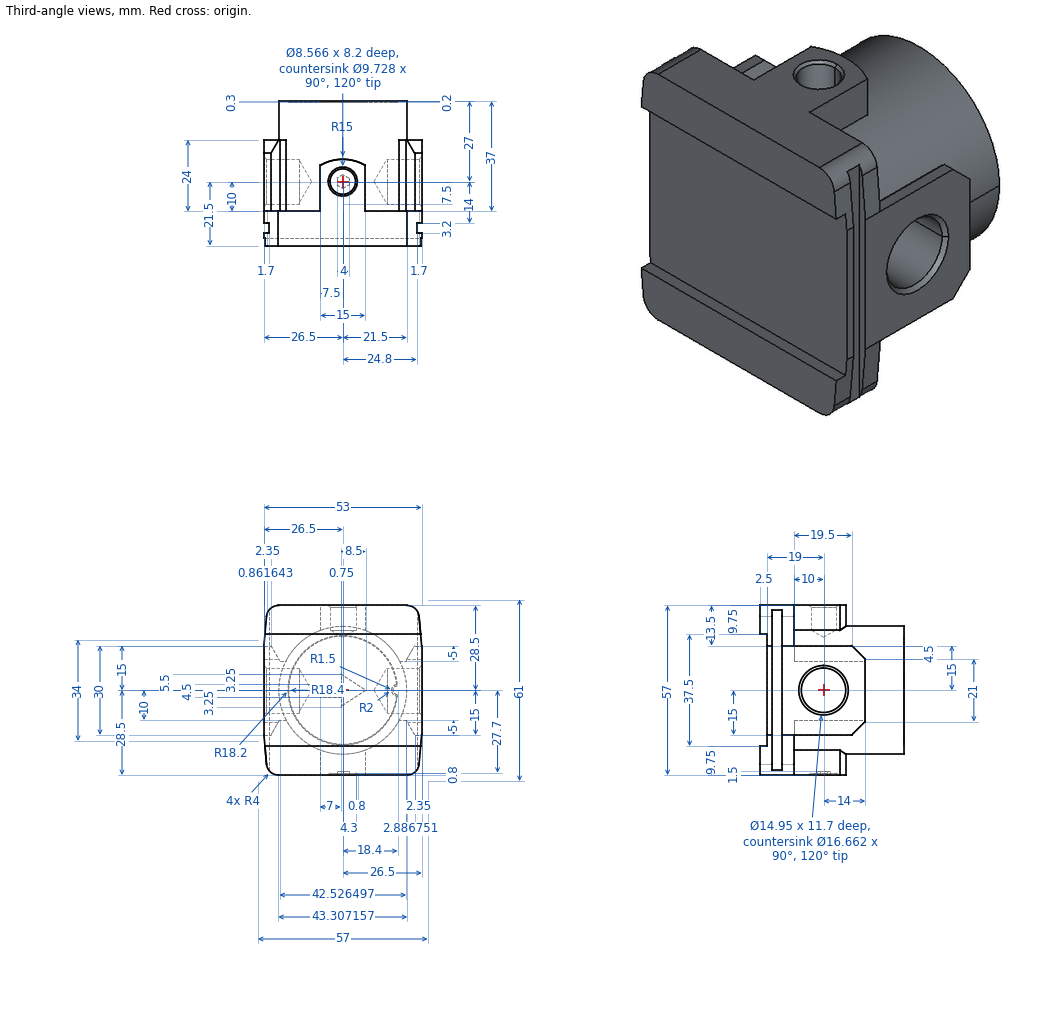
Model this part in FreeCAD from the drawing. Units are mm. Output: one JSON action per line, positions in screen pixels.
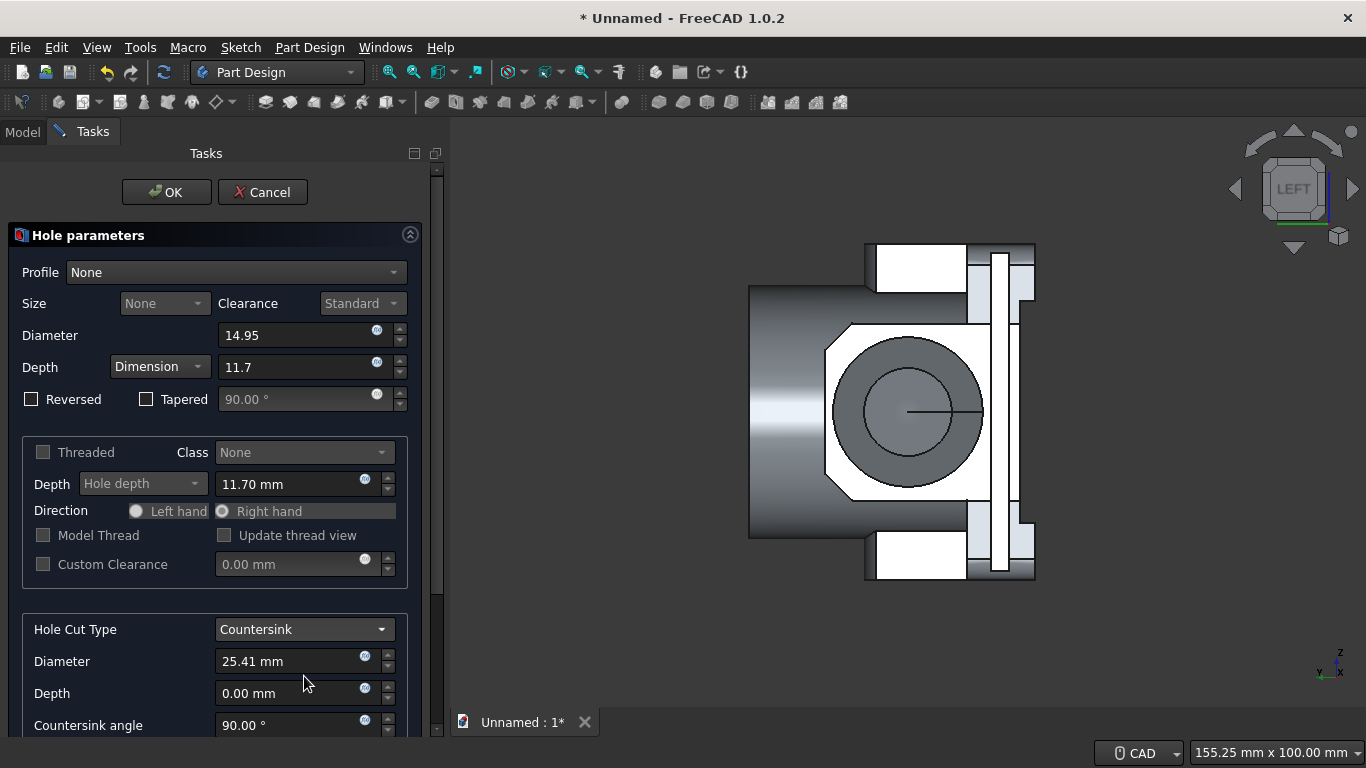
{"action": "triple_click", "coordinate": [298, 661]}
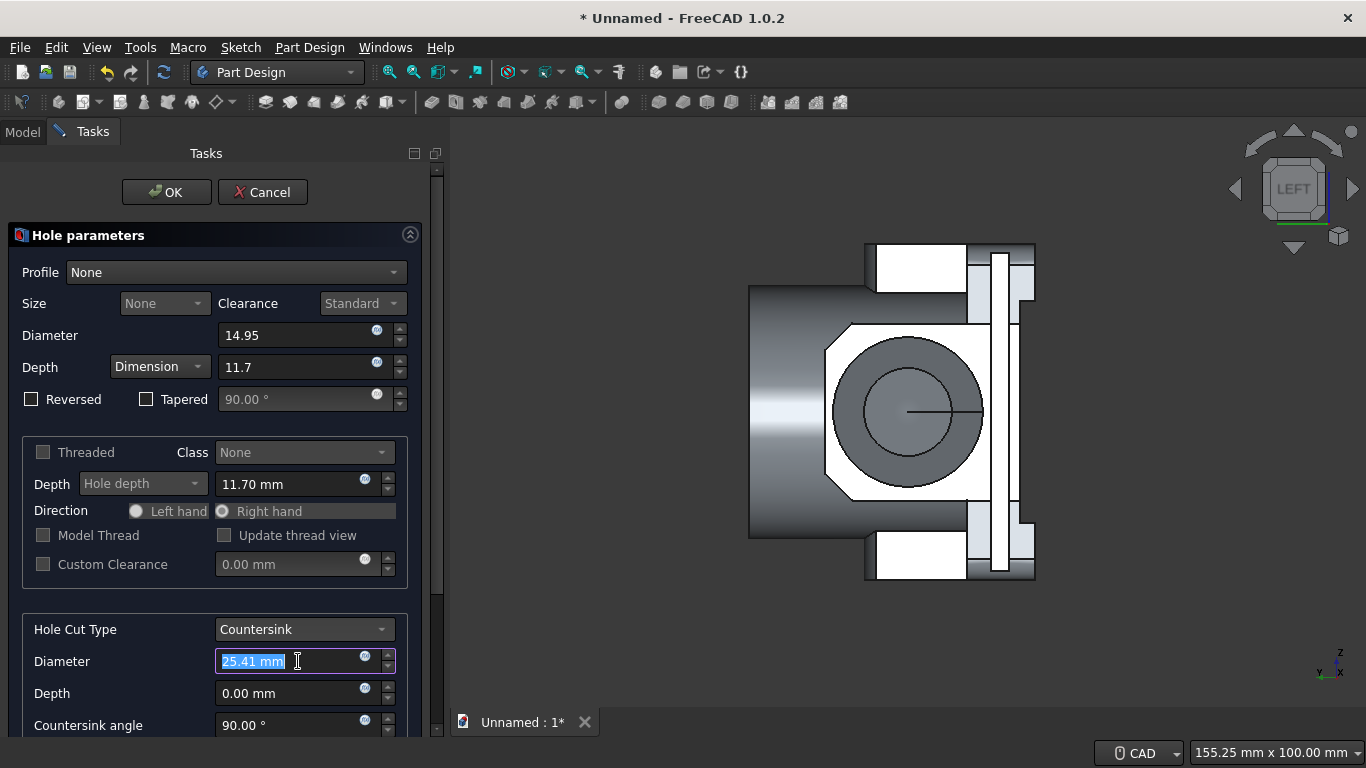
{"action": "type", "text": "16.662"}
{"action": "key", "text": "Tab"}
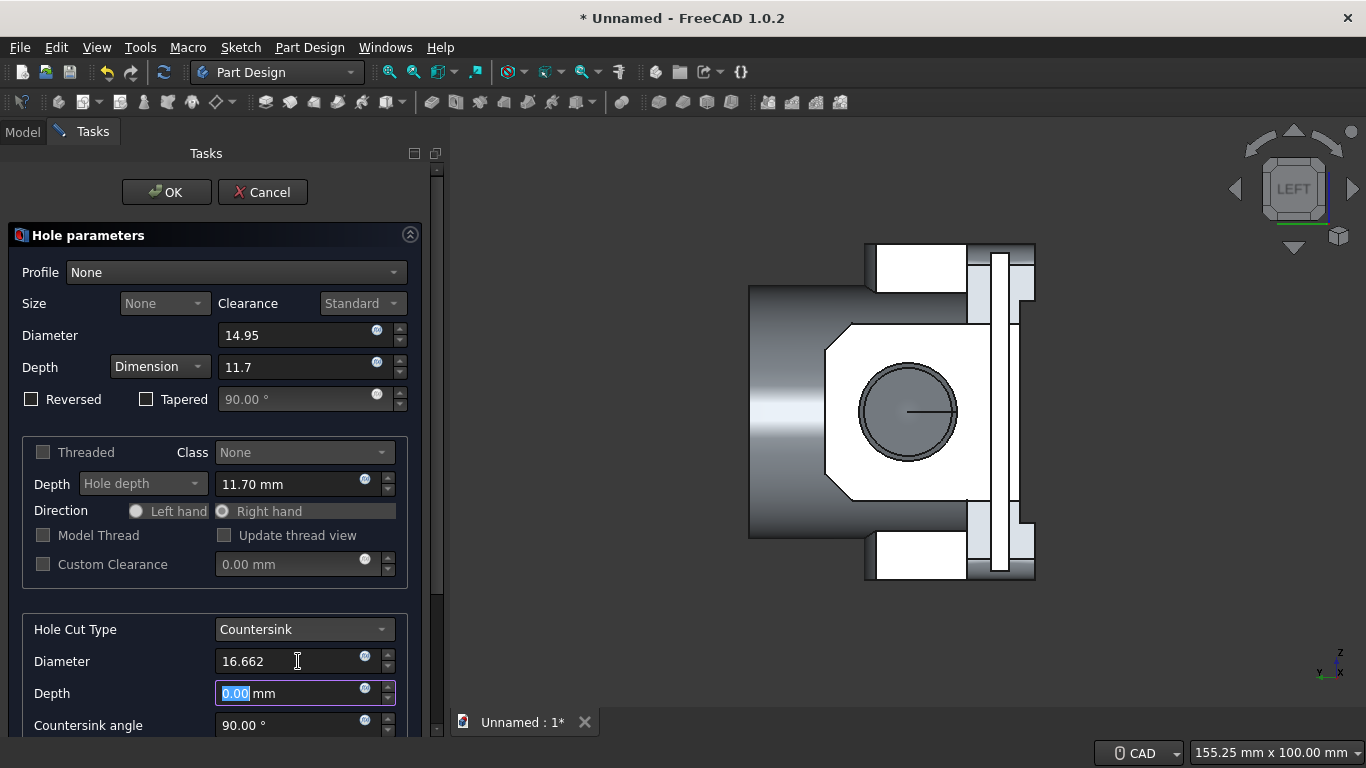
{"action": "scroll", "coordinate": [437, 450], "scroll_direction": "down", "scroll_amount": 3}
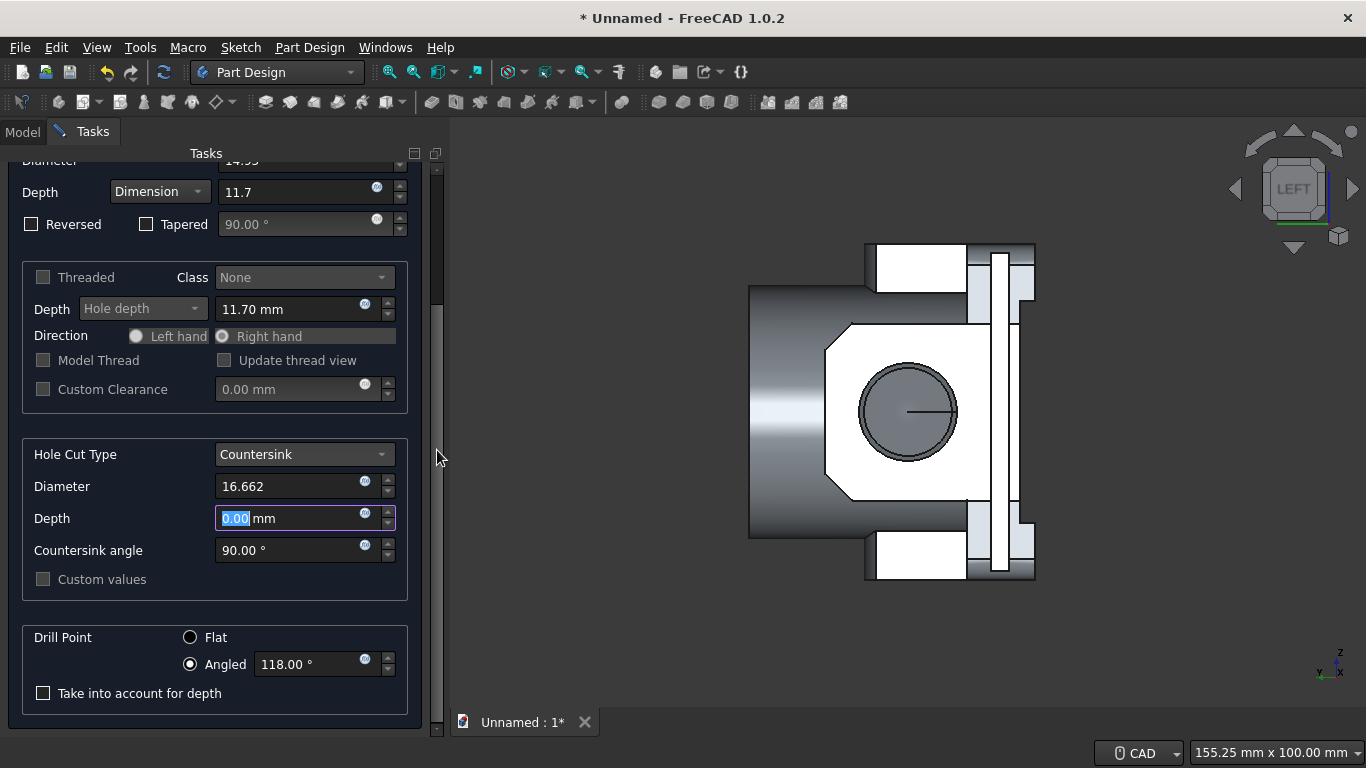
{"action": "triple_click", "coordinate": [317, 664]}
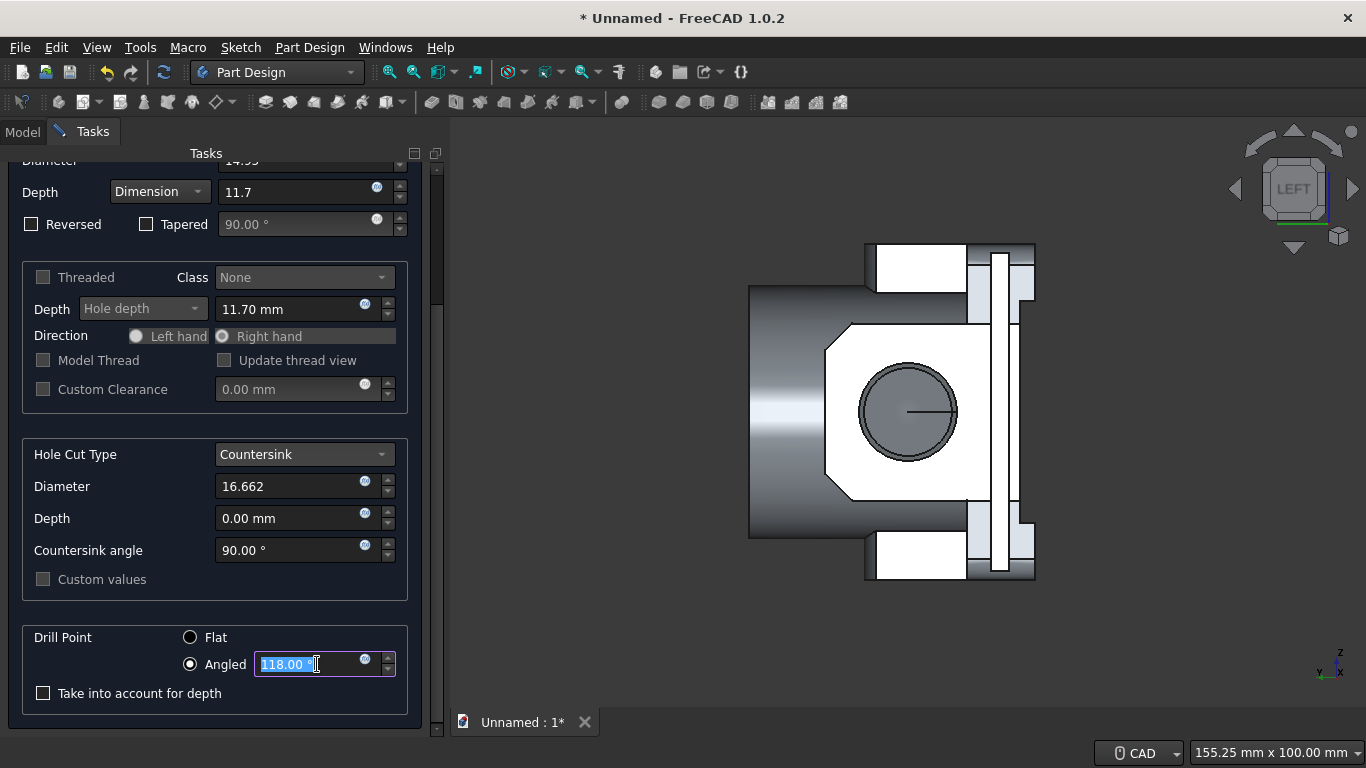
{"action": "type", "text": "120"}
{"action": "key", "text": "Tab"}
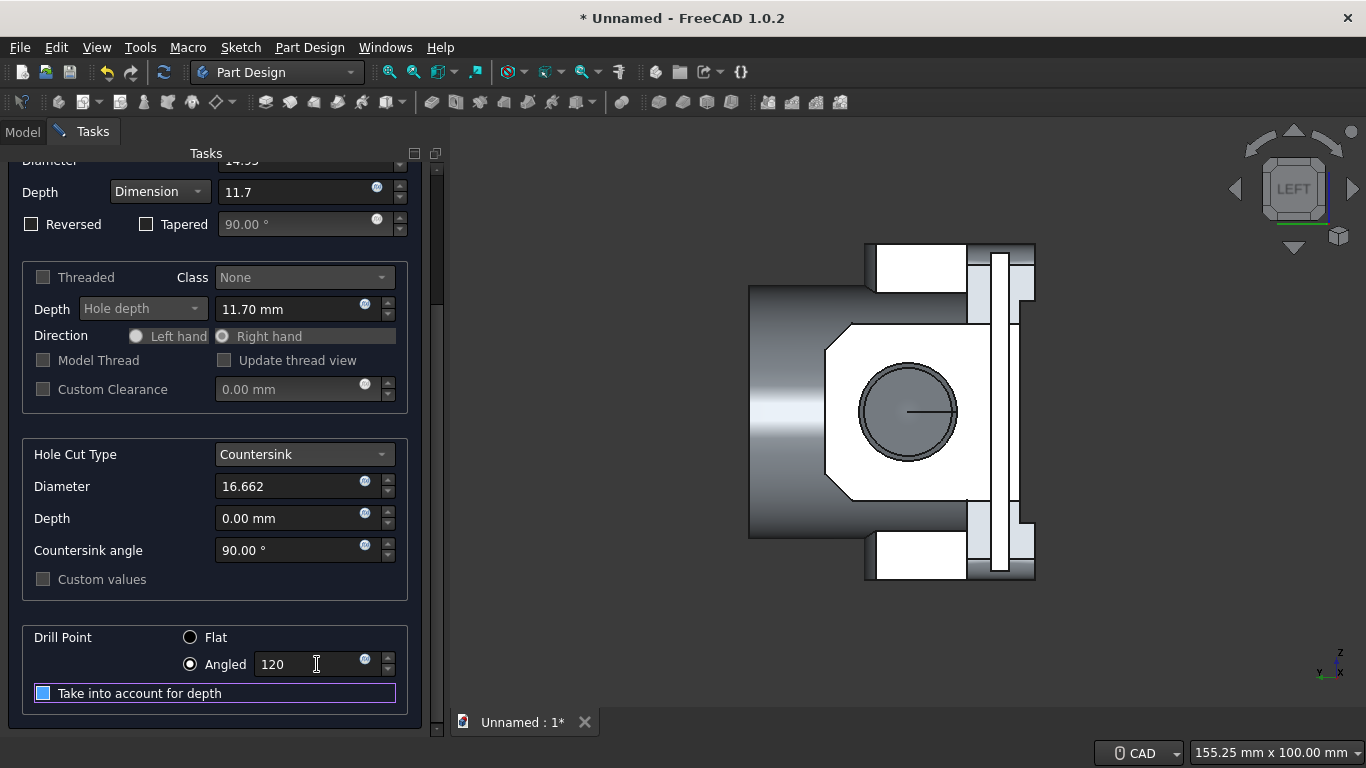
{"action": "scroll", "coordinate": [437, 450], "scroll_direction": "up", "scroll_amount": 4}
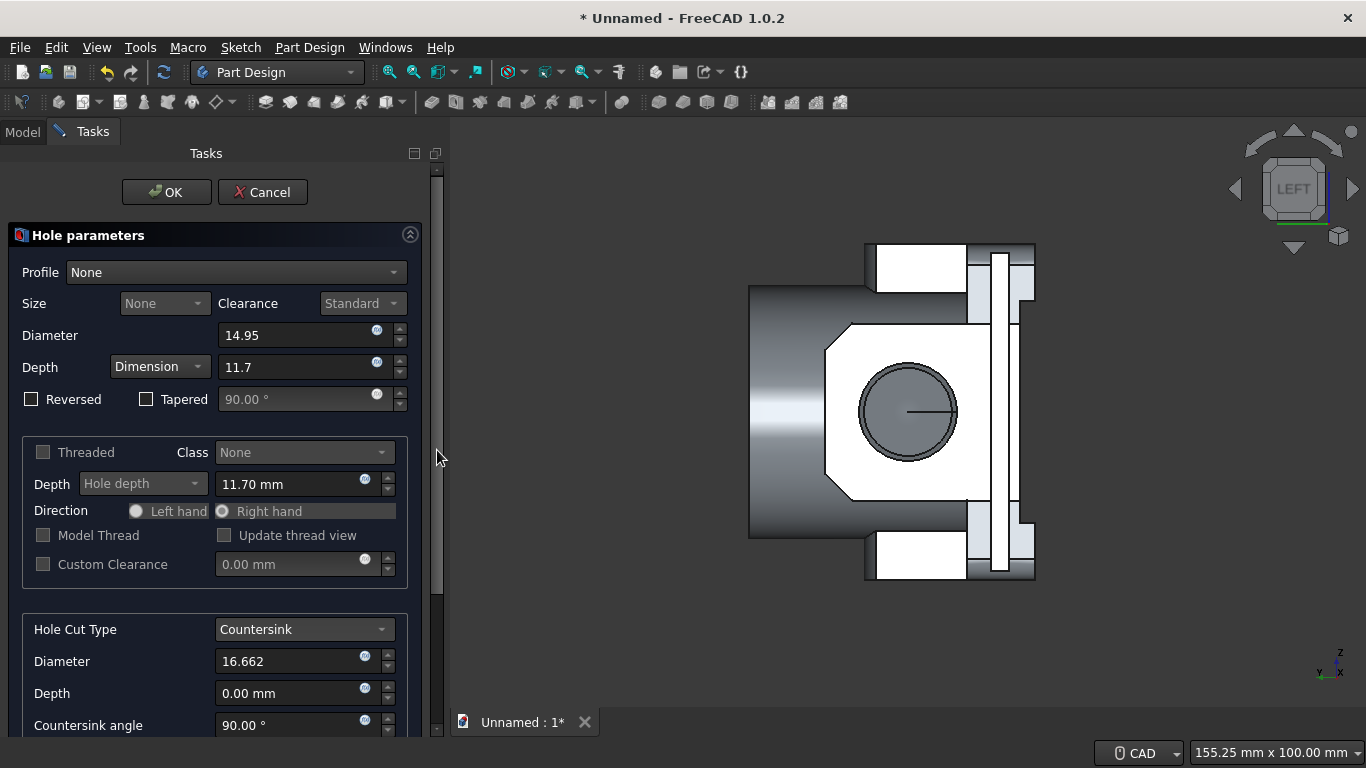
{"action": "left_click", "coordinate": [167, 192]}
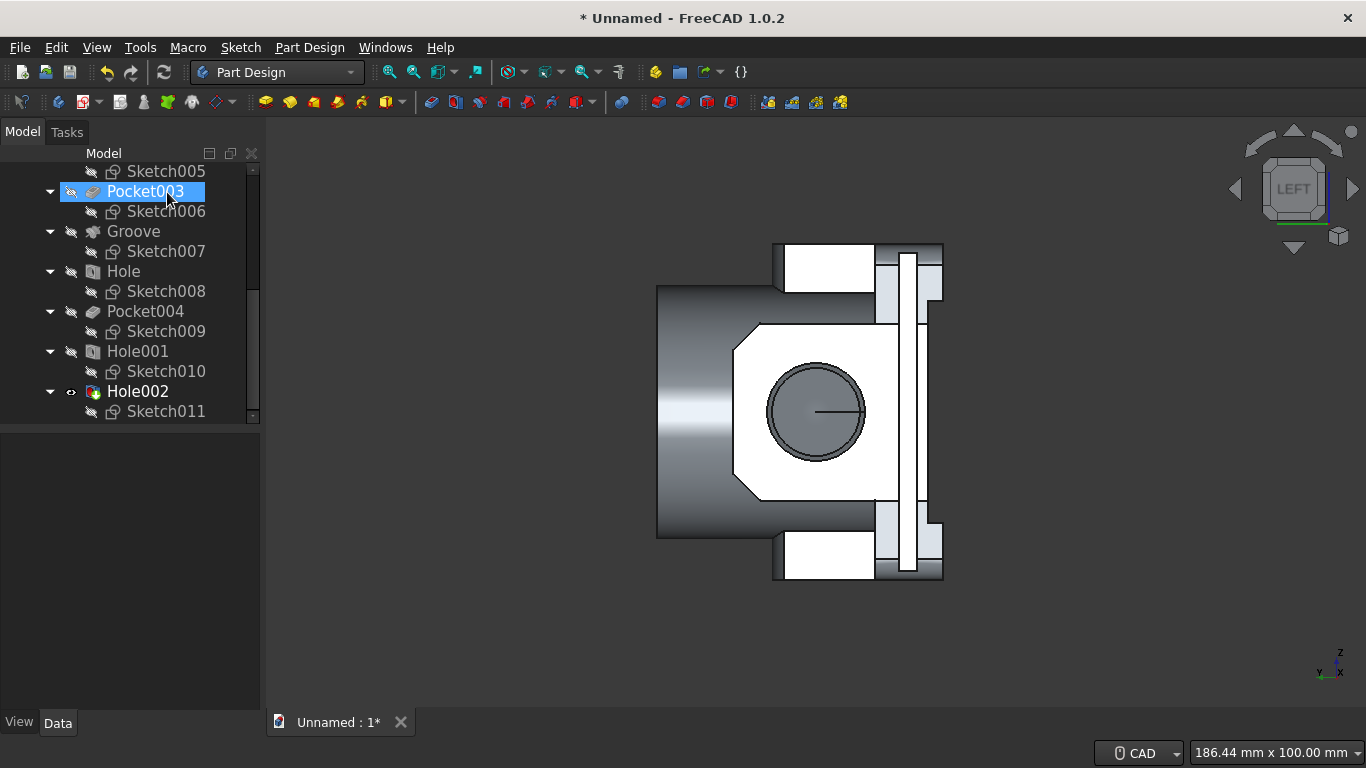
{"action": "key", "text": "4"}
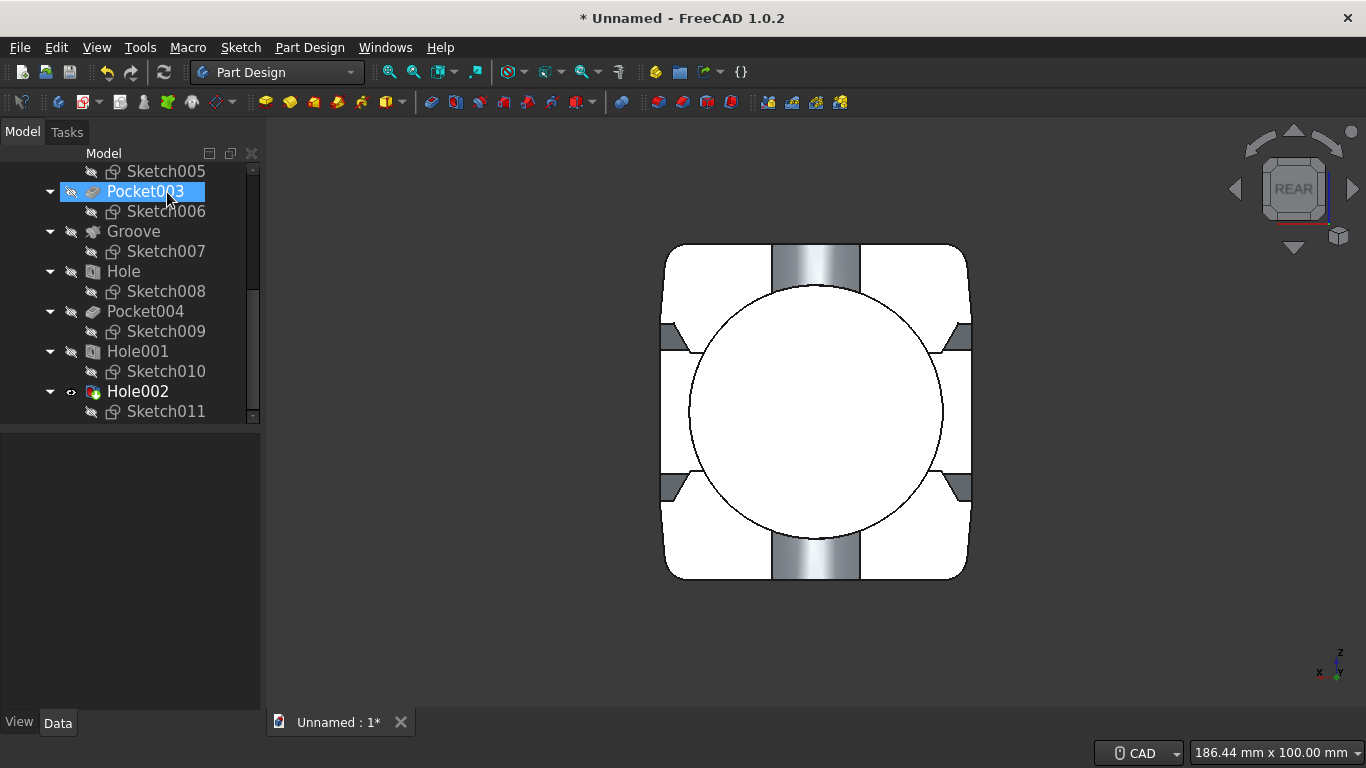
{"action": "left_click", "coordinate": [816, 411]}